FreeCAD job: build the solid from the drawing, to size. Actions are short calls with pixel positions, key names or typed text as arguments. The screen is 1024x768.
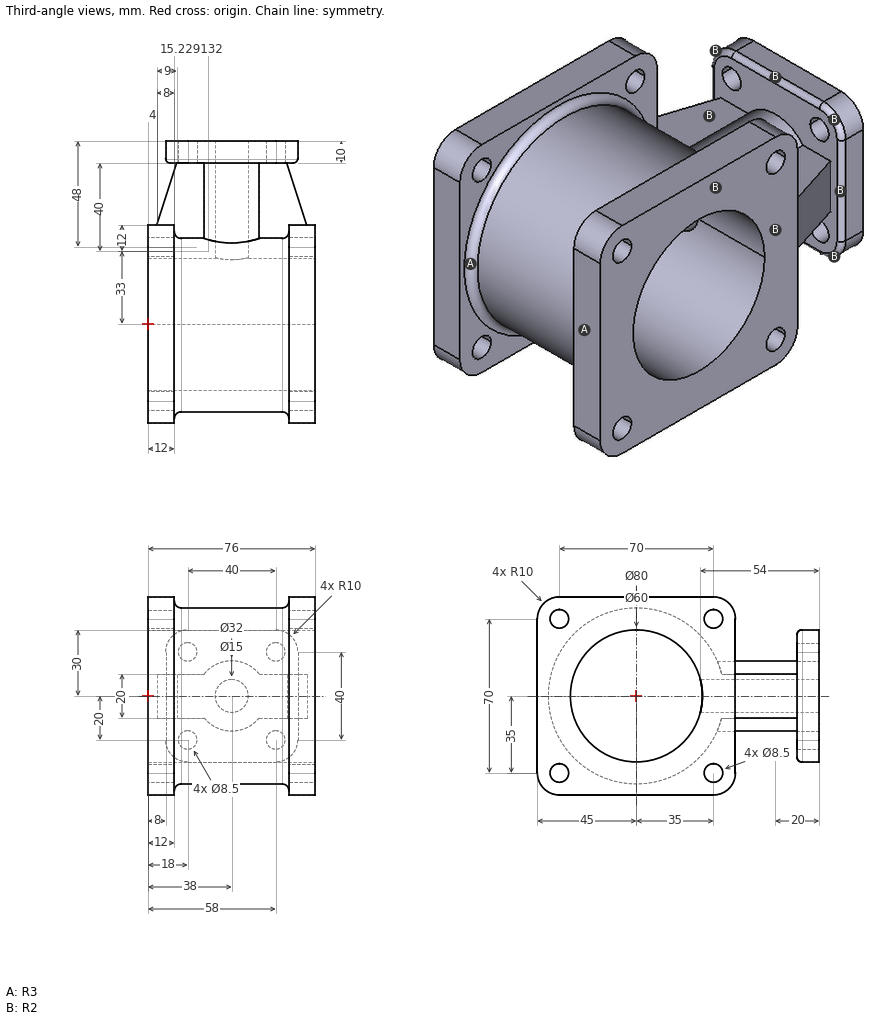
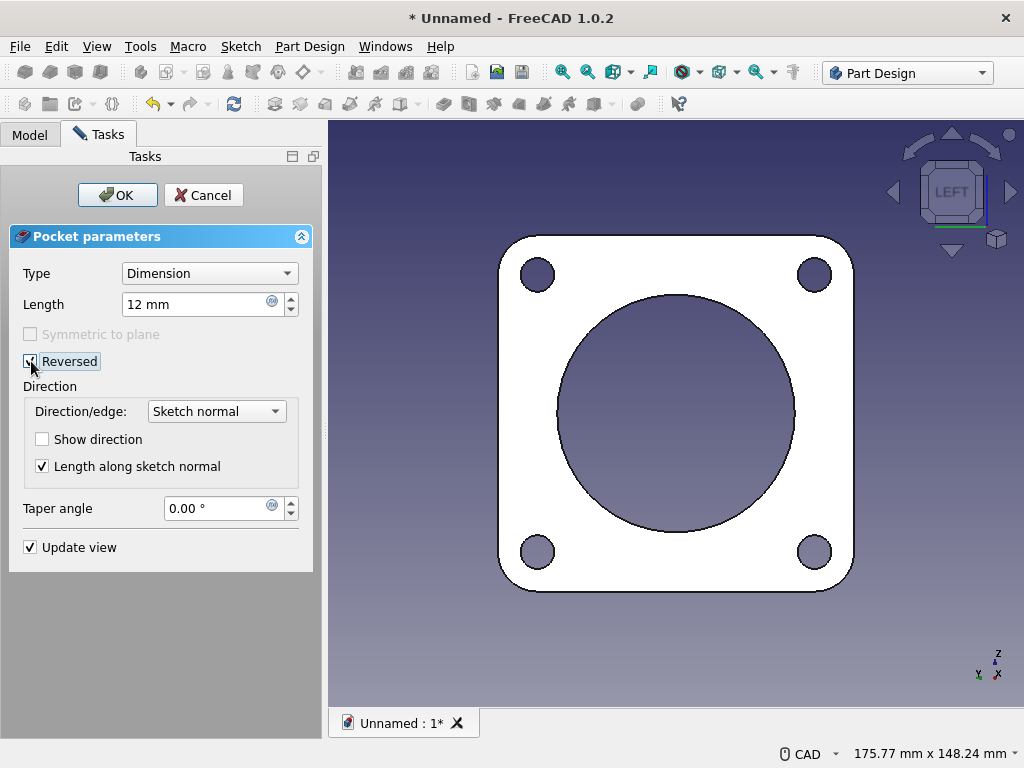
click(118, 195)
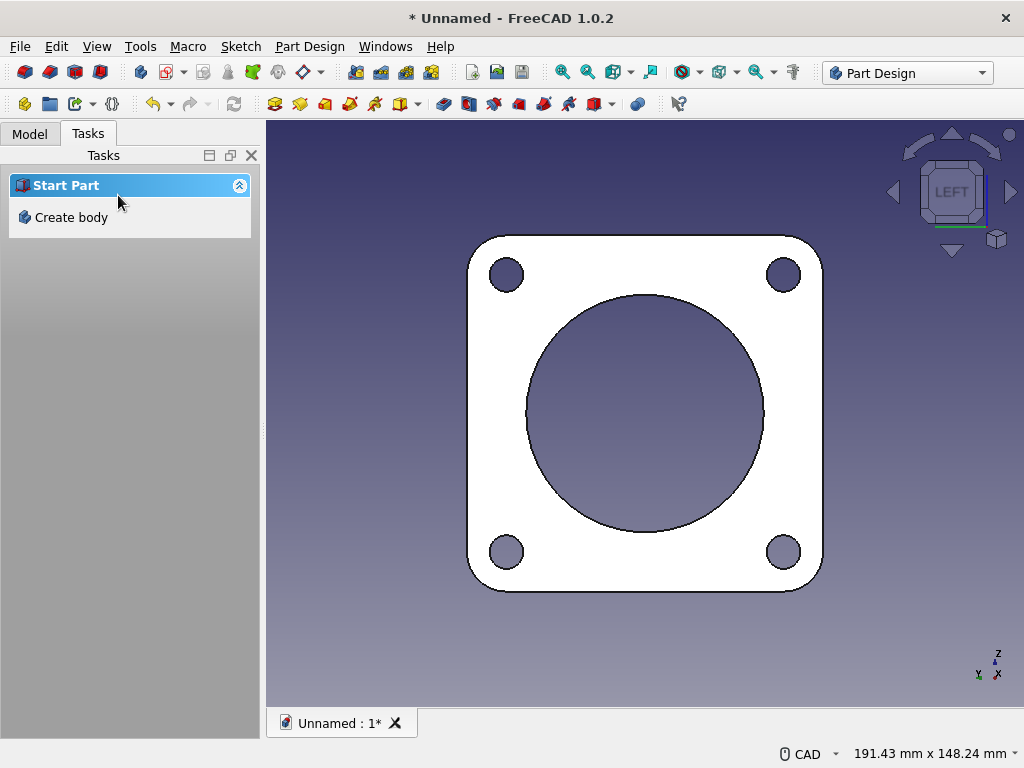
click(30, 134)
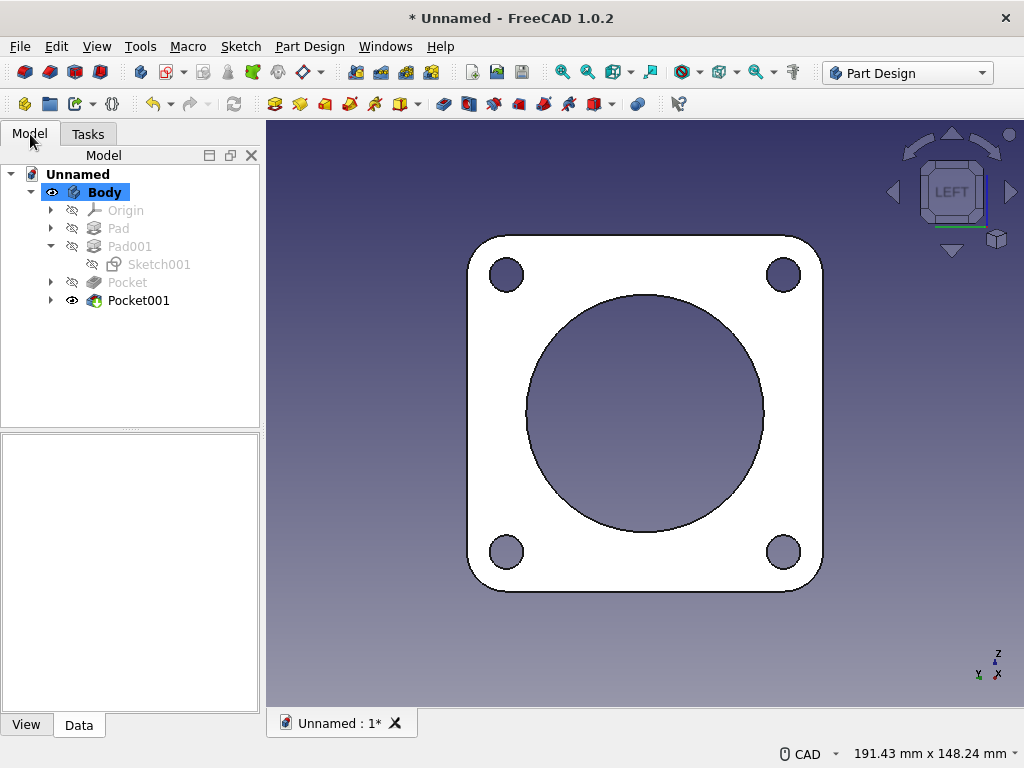
click(51, 210)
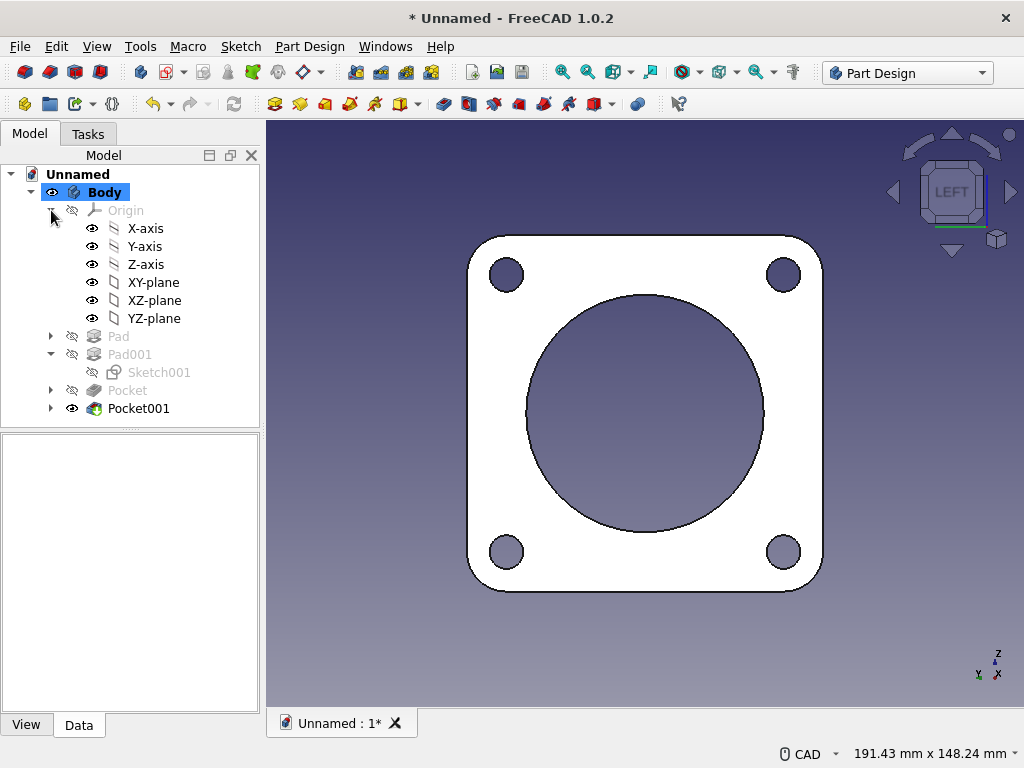
click(137, 318)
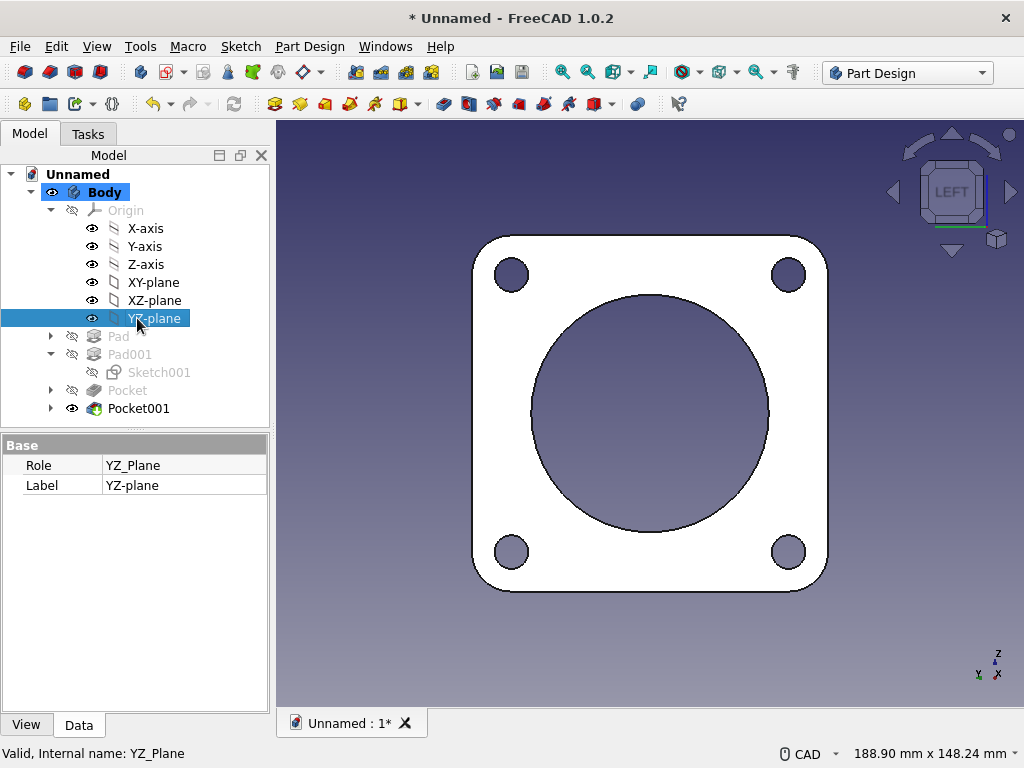
click(302, 72)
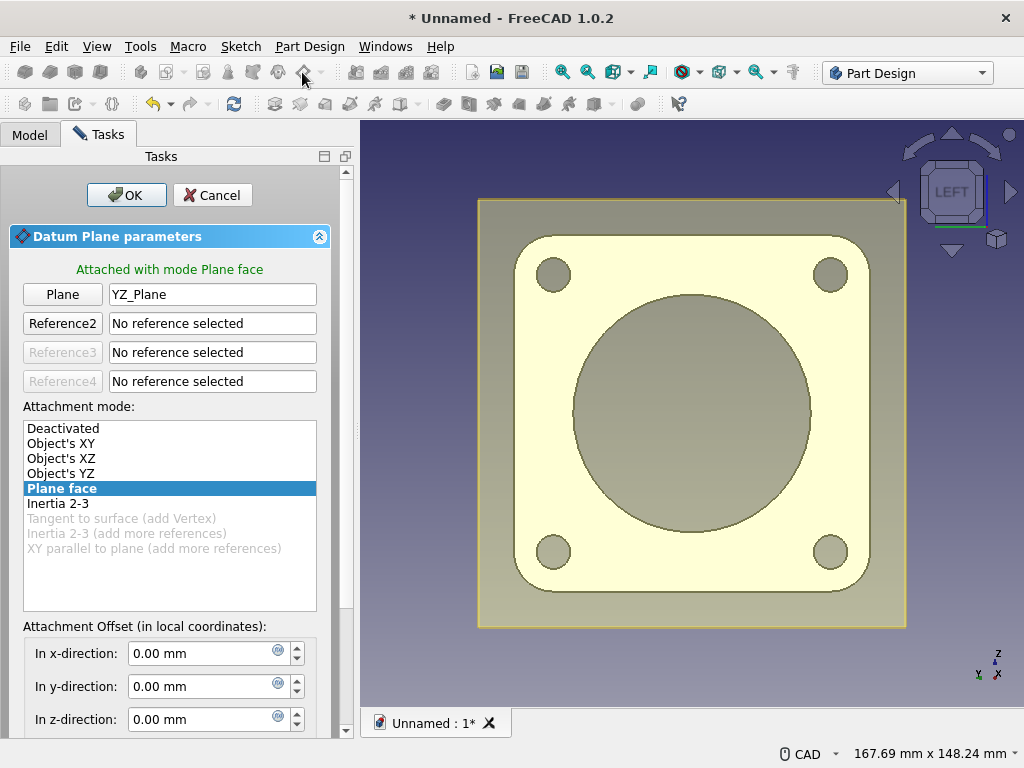
triple_click(210, 720)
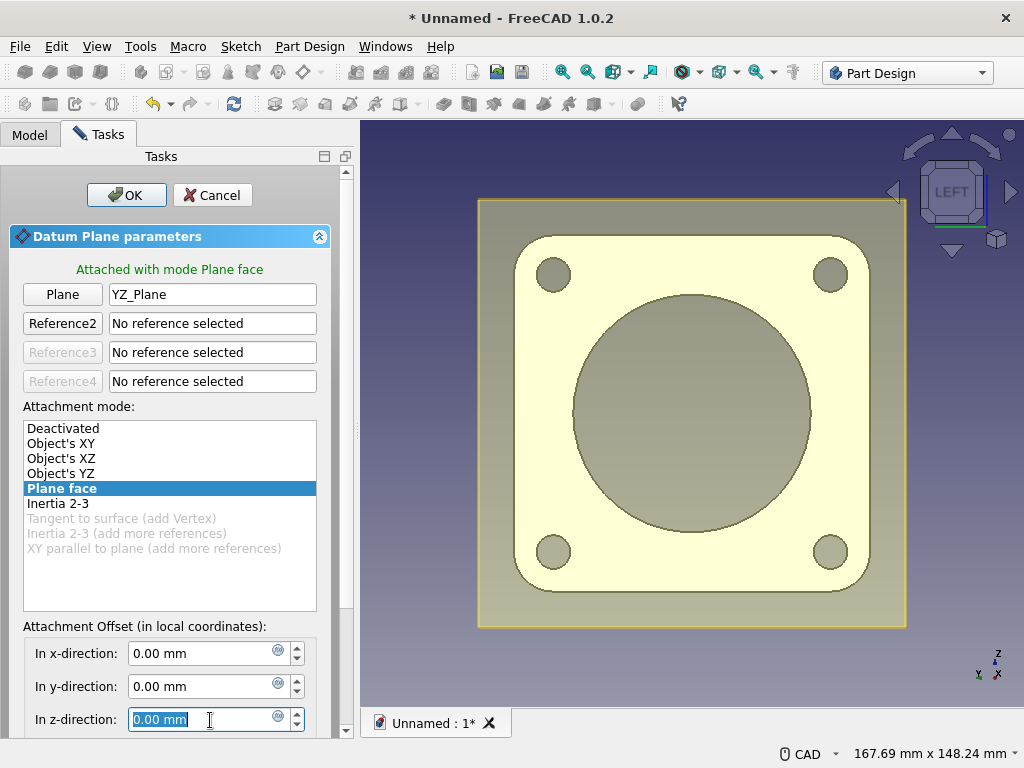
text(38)
key(Tab)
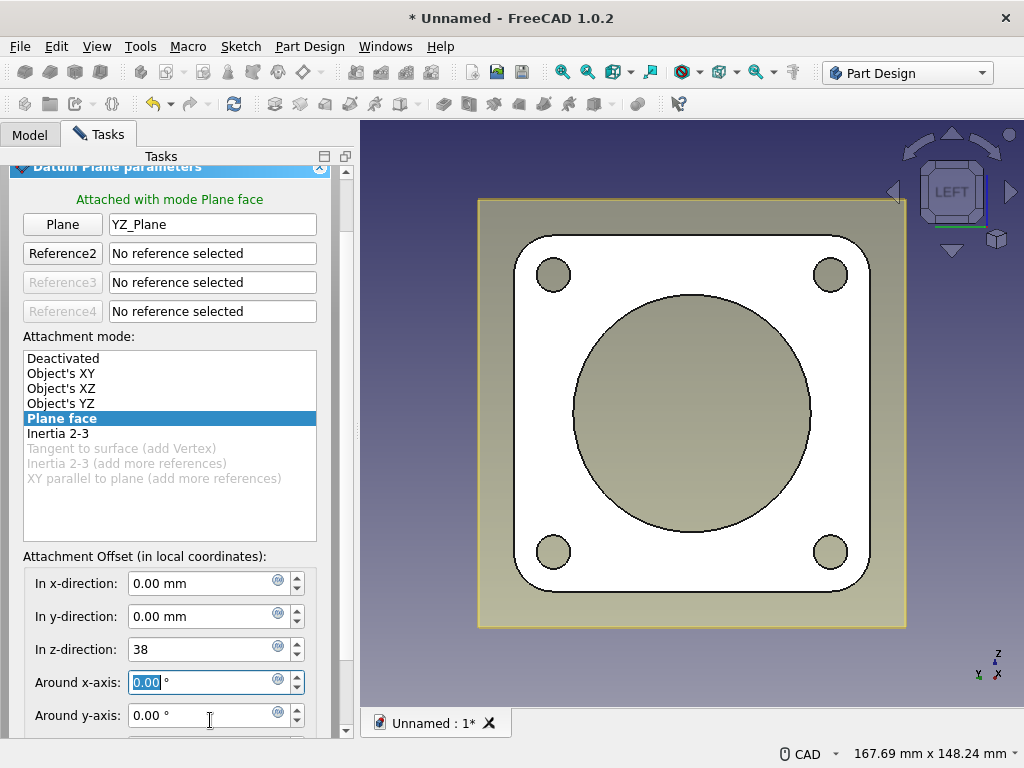
scroll(346, 452, up, 2)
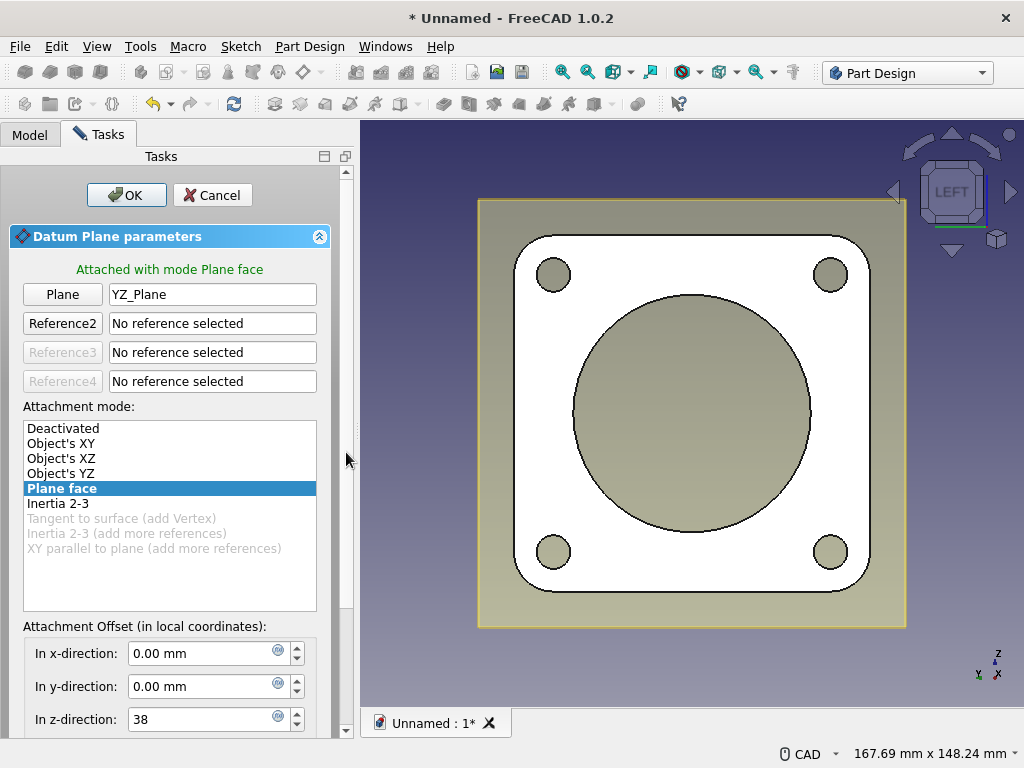
click(127, 195)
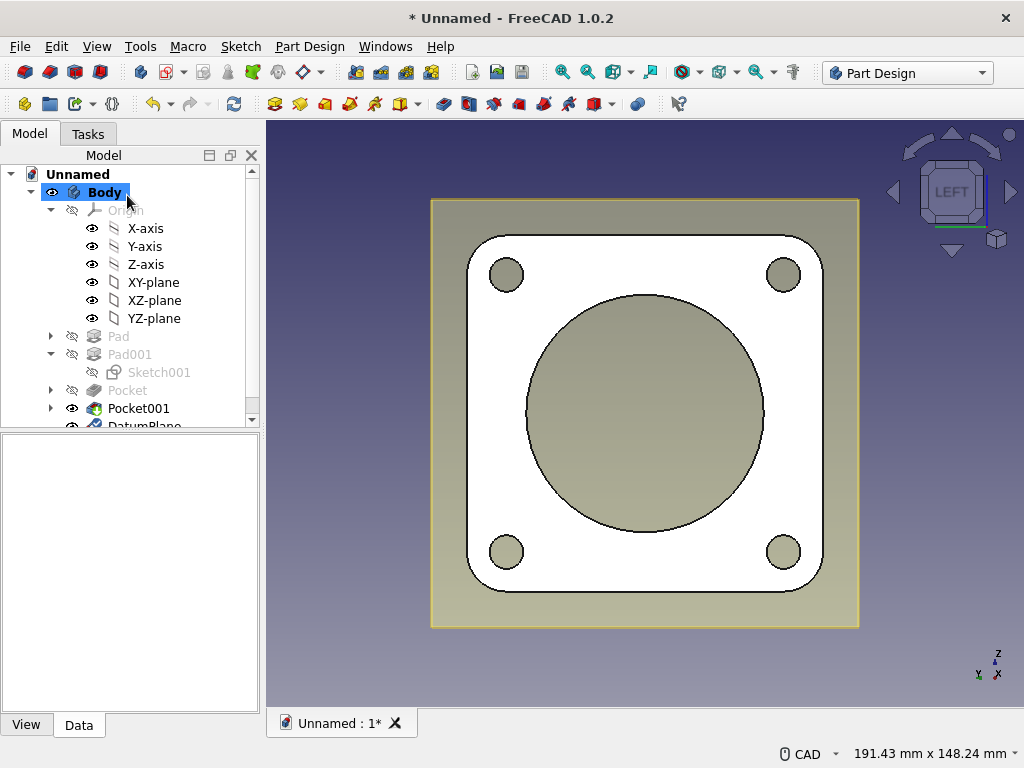
click(117, 354)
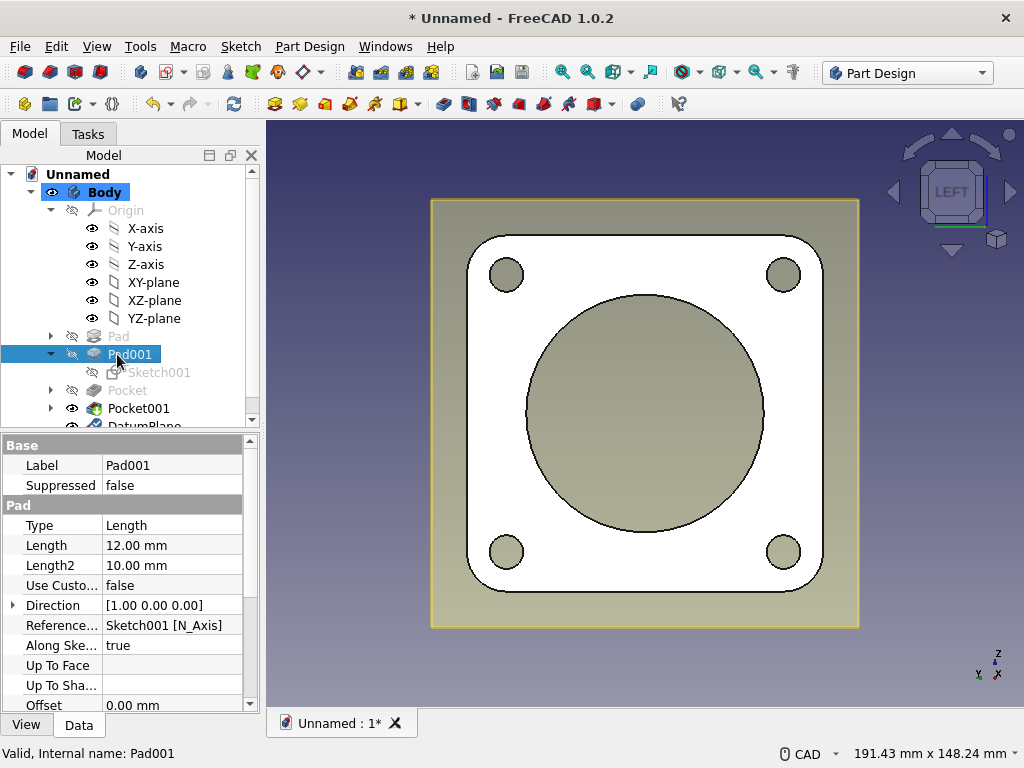
click(356, 72)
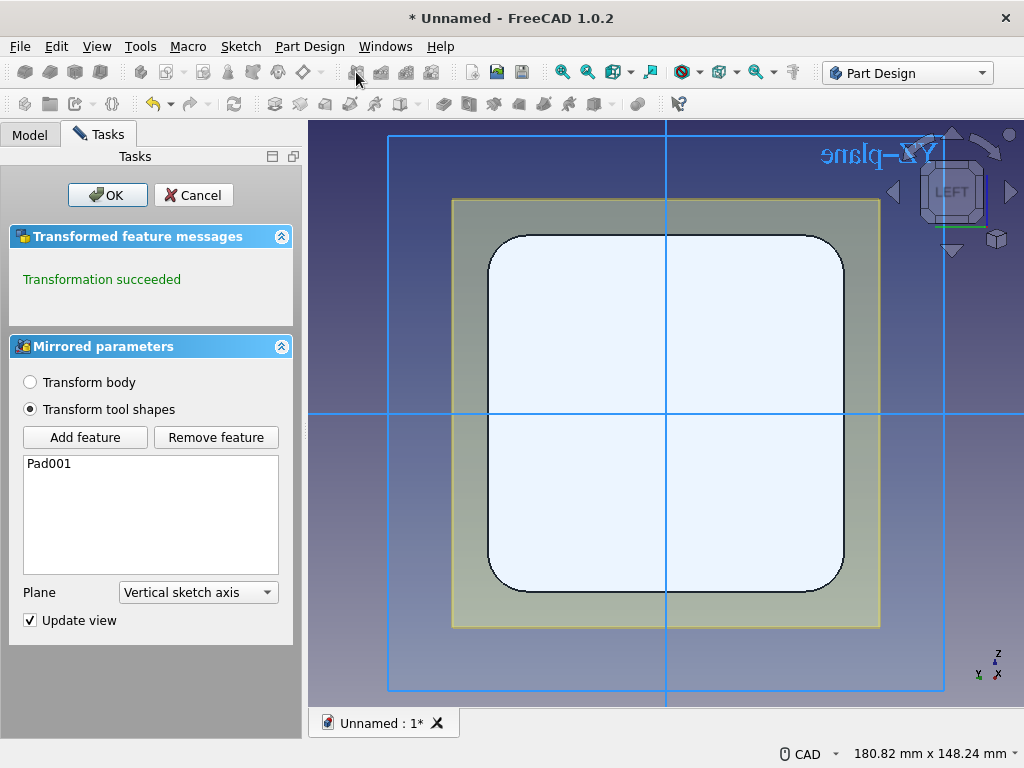
click(199, 592)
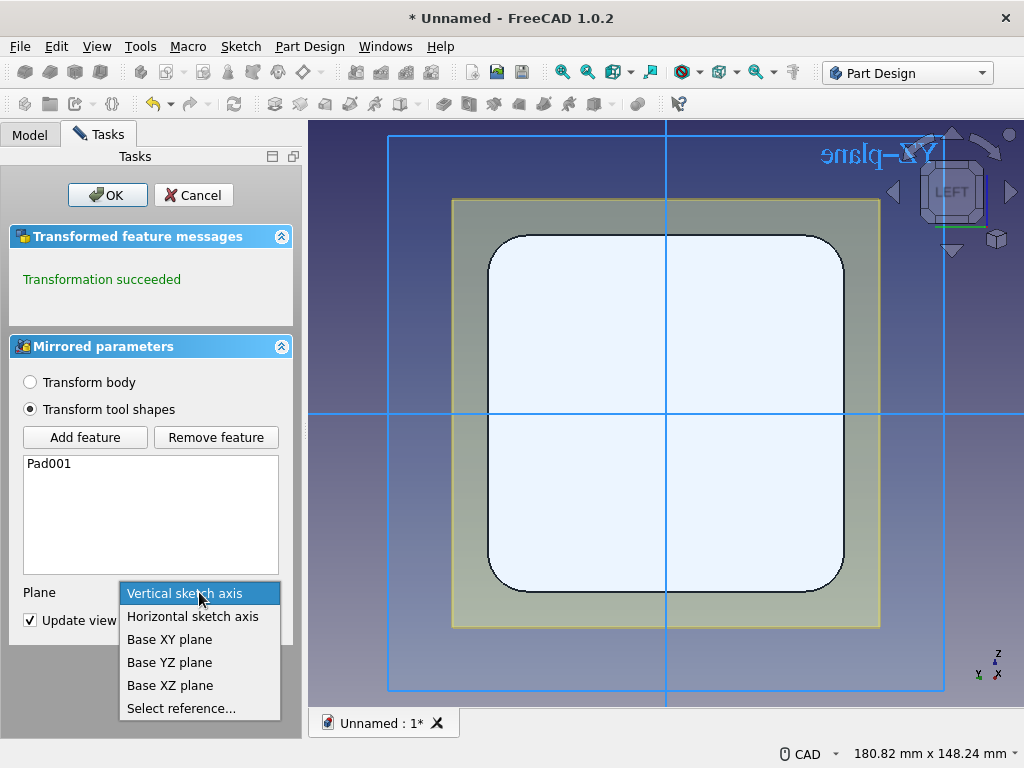
click(198, 708)